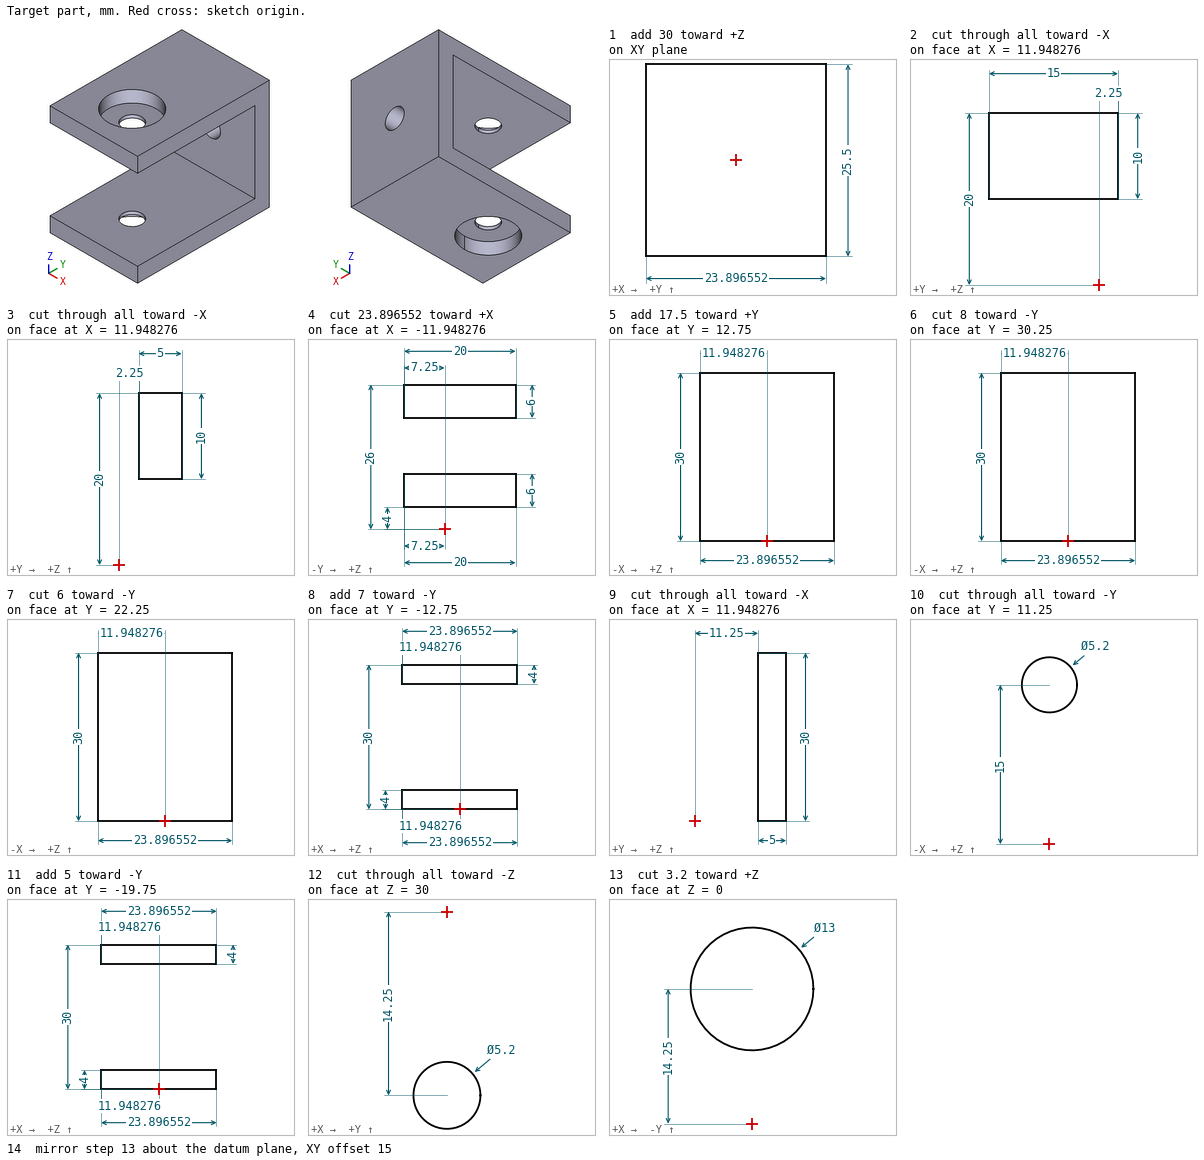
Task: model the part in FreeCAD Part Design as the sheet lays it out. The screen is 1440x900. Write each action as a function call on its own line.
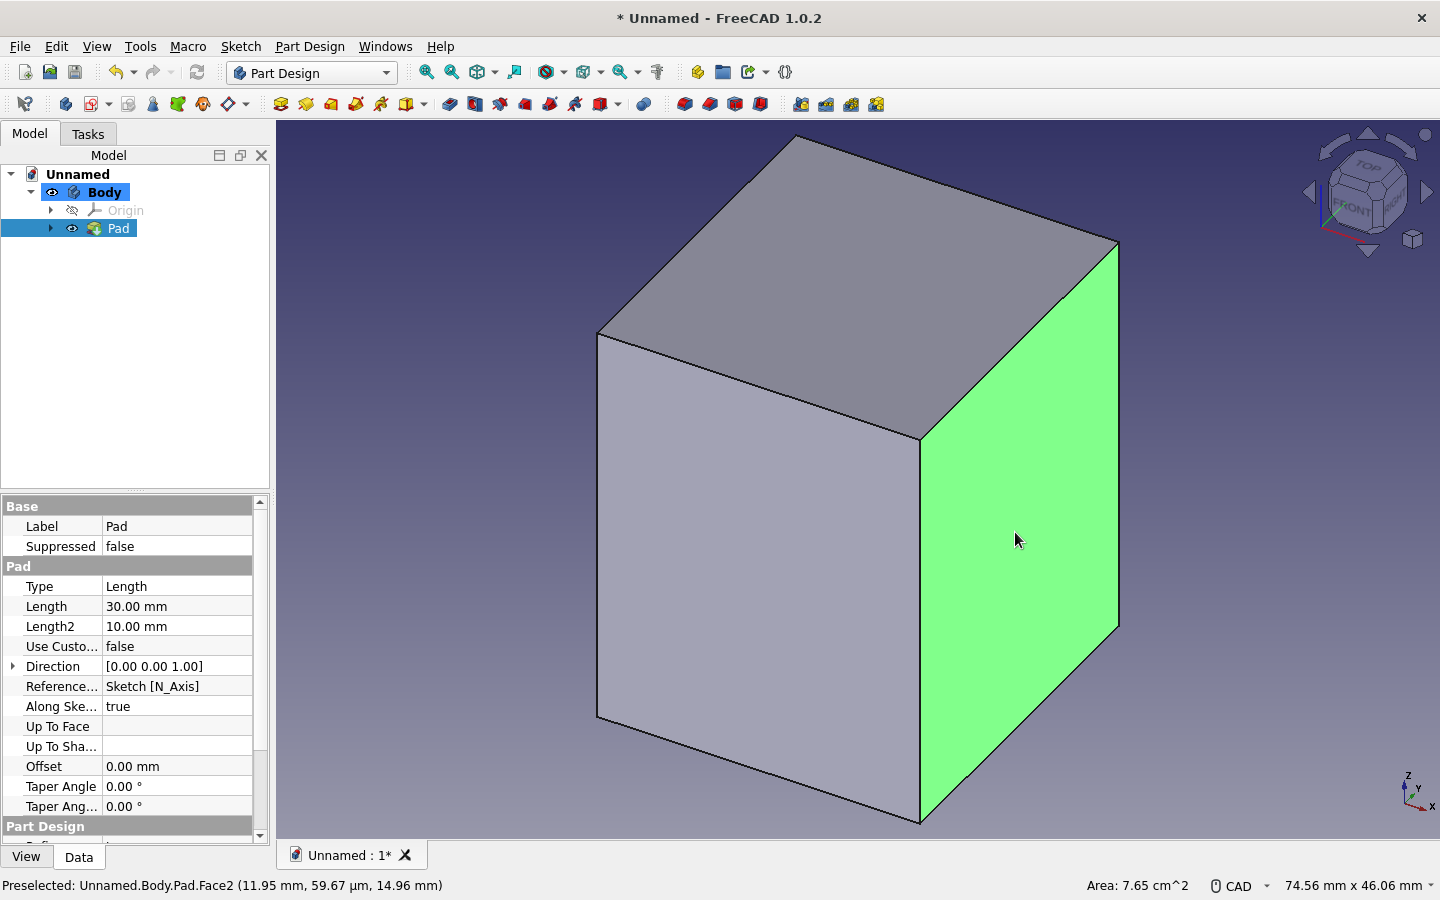
click(90, 104)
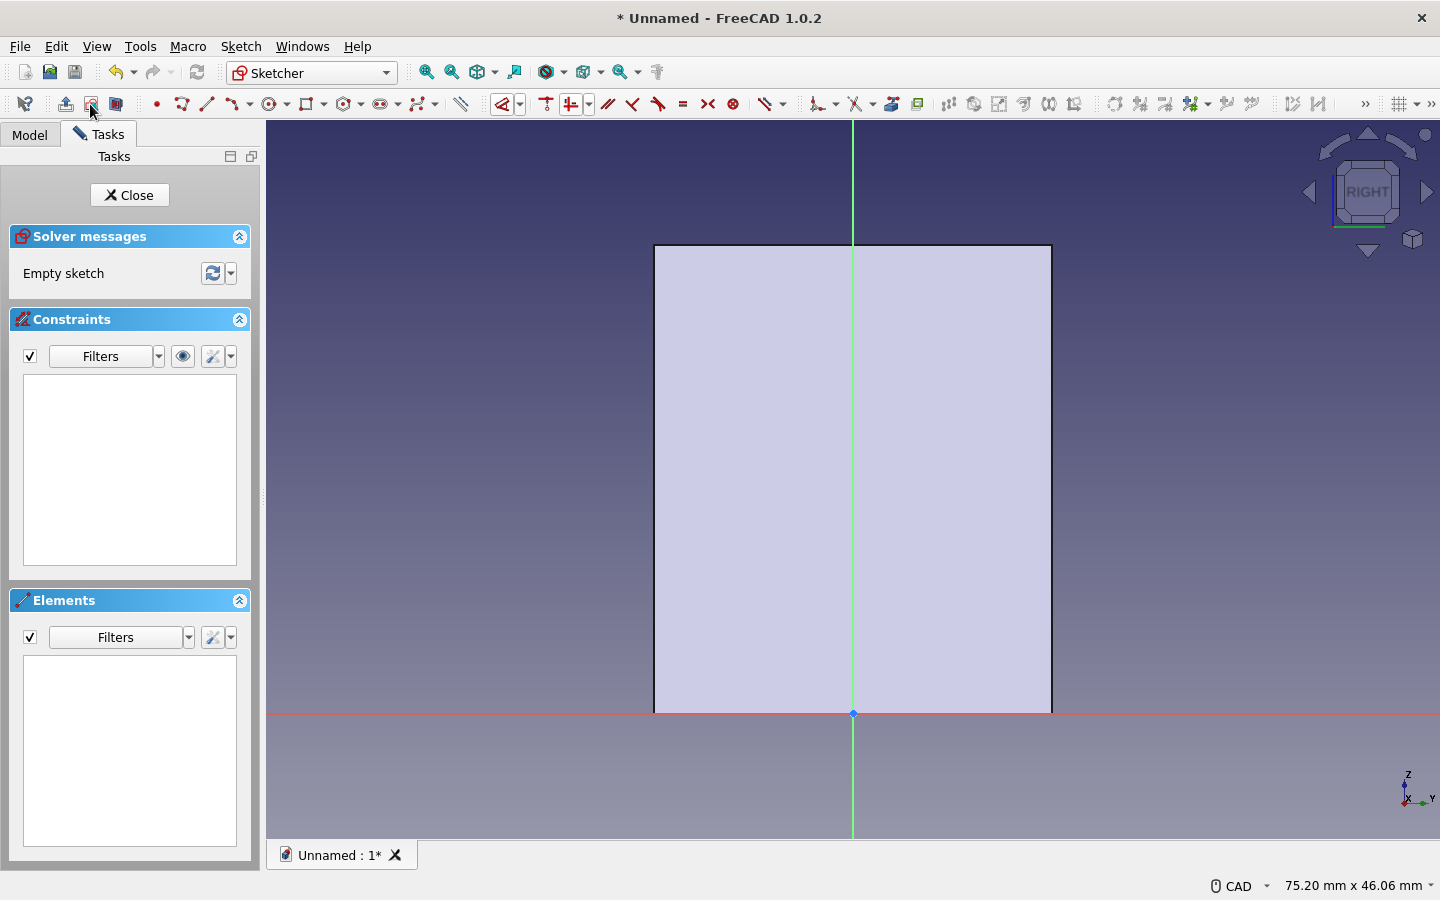
scroll(744, 716, up, 2)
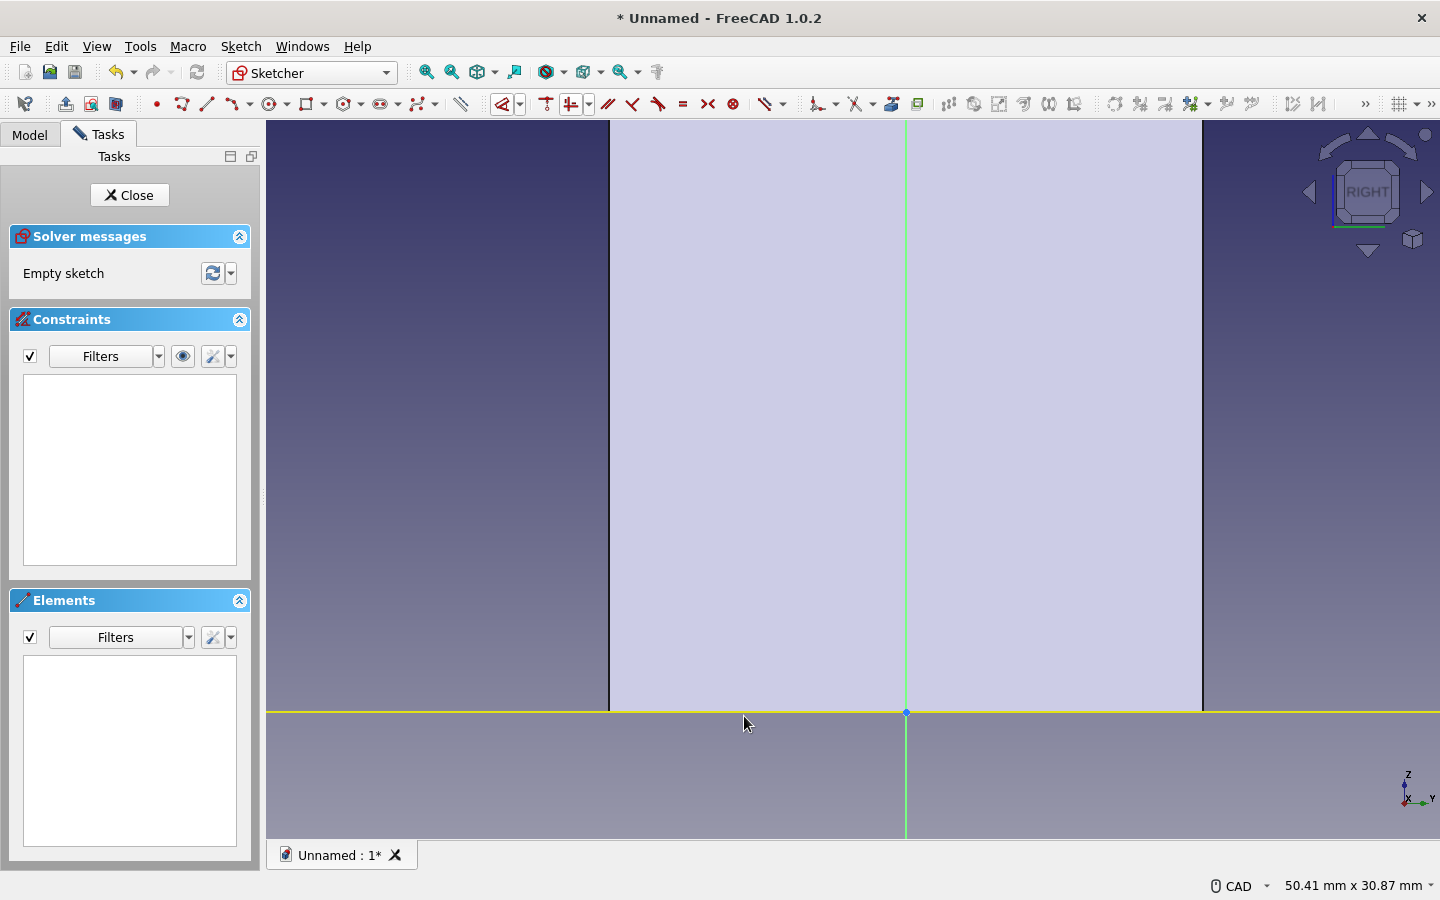
click(306, 104)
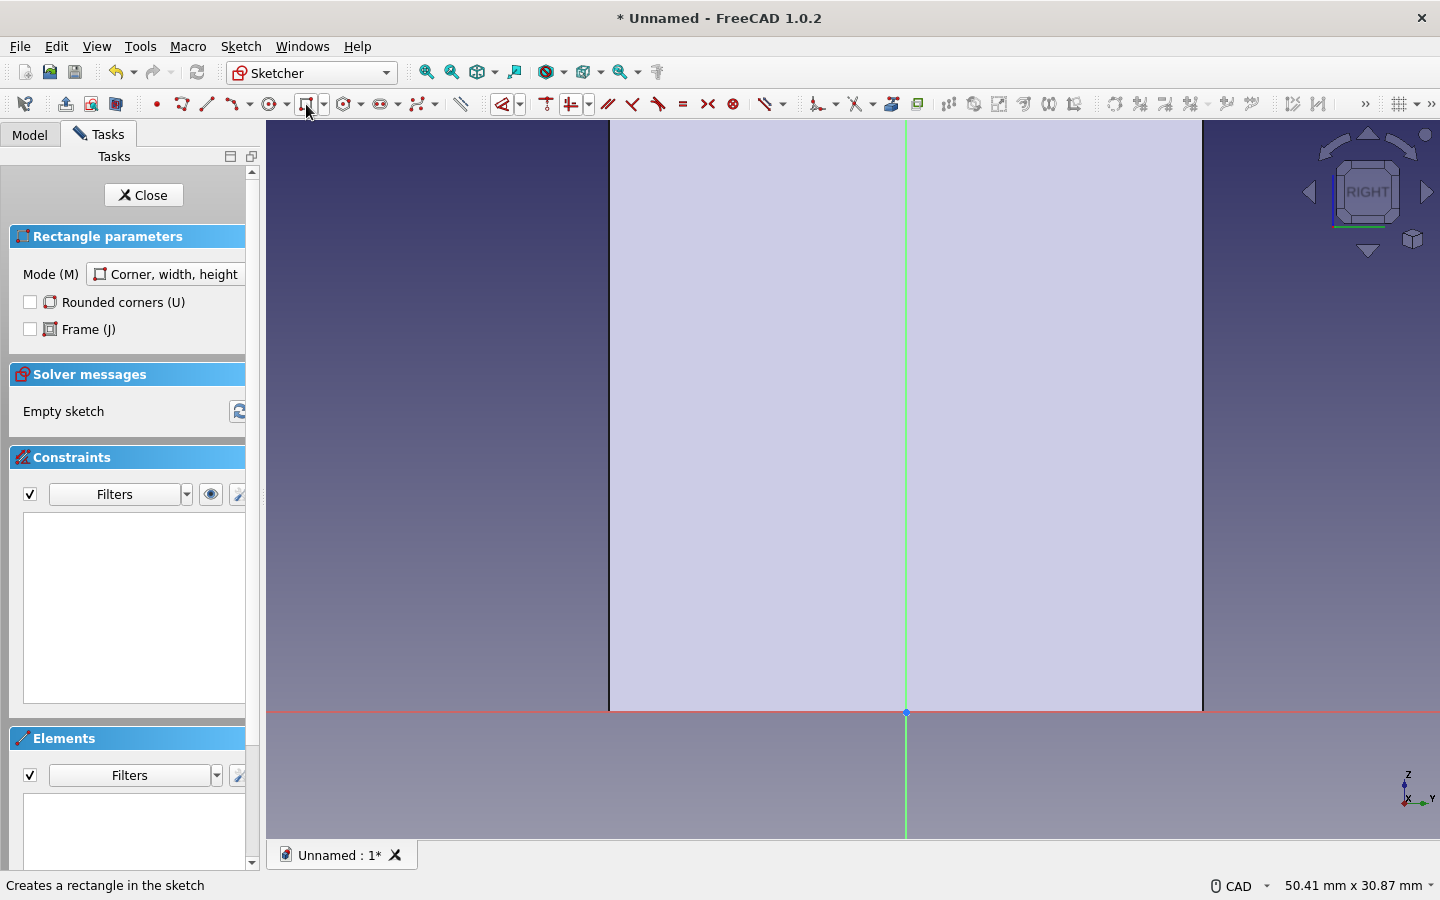
click(609, 246)
move(959, 479)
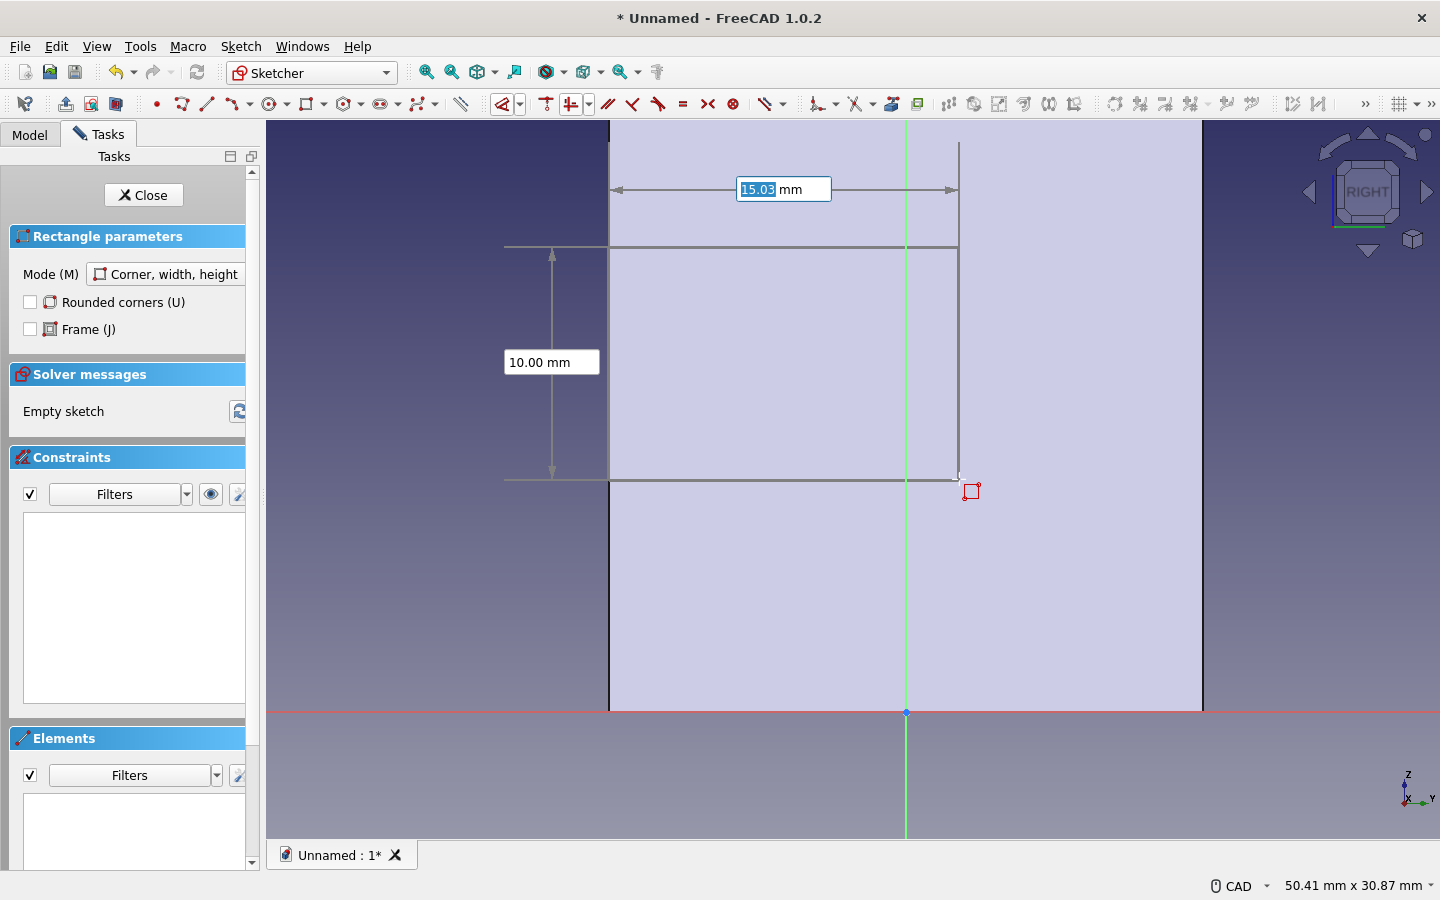
text(15)
key(Tab)
text(10)
key(Return)
key(Escape)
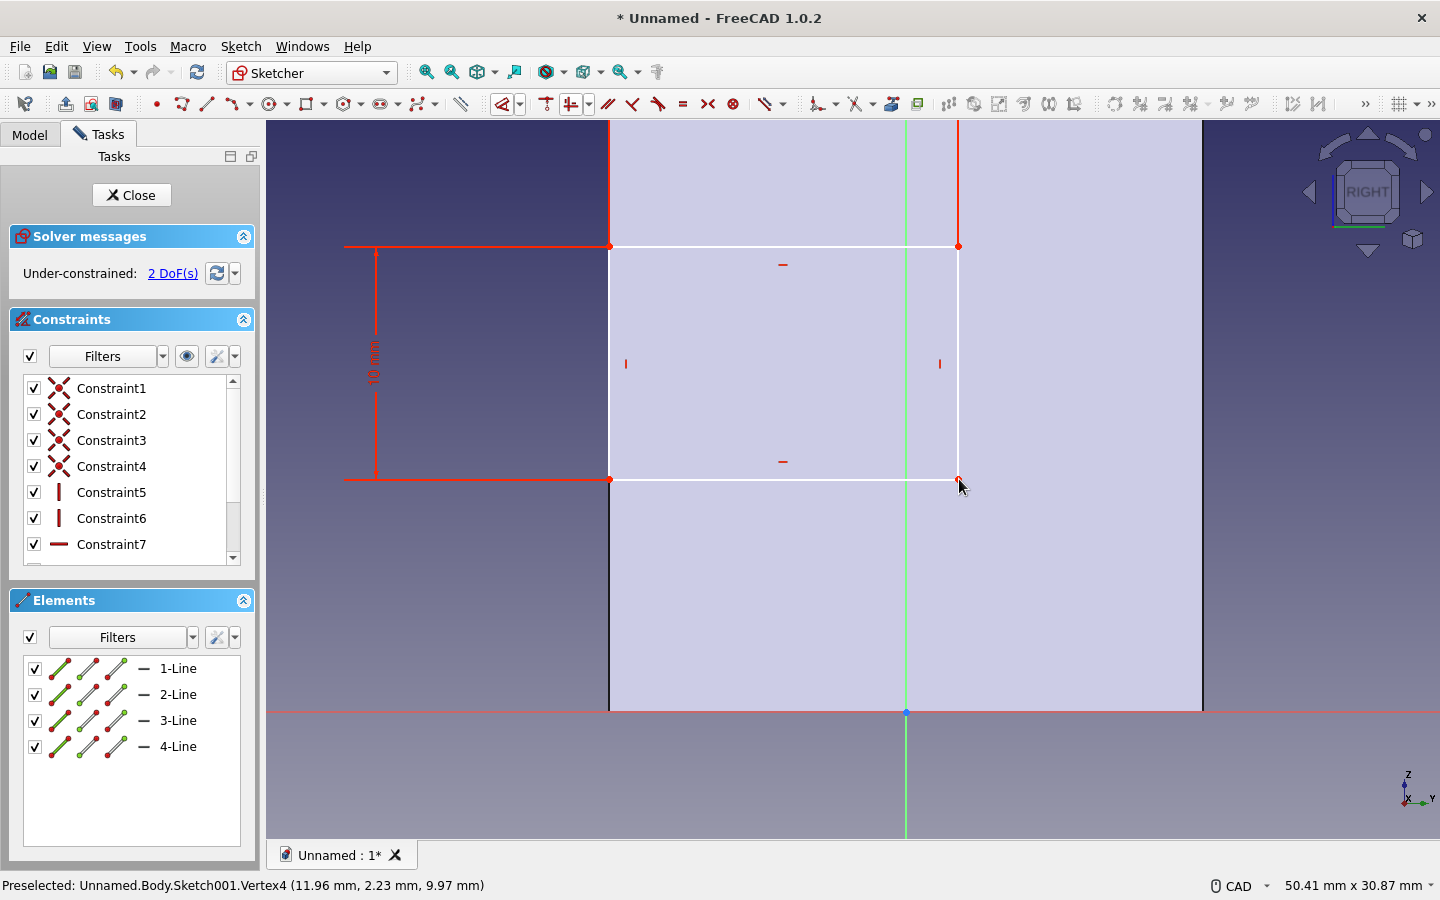
key(d)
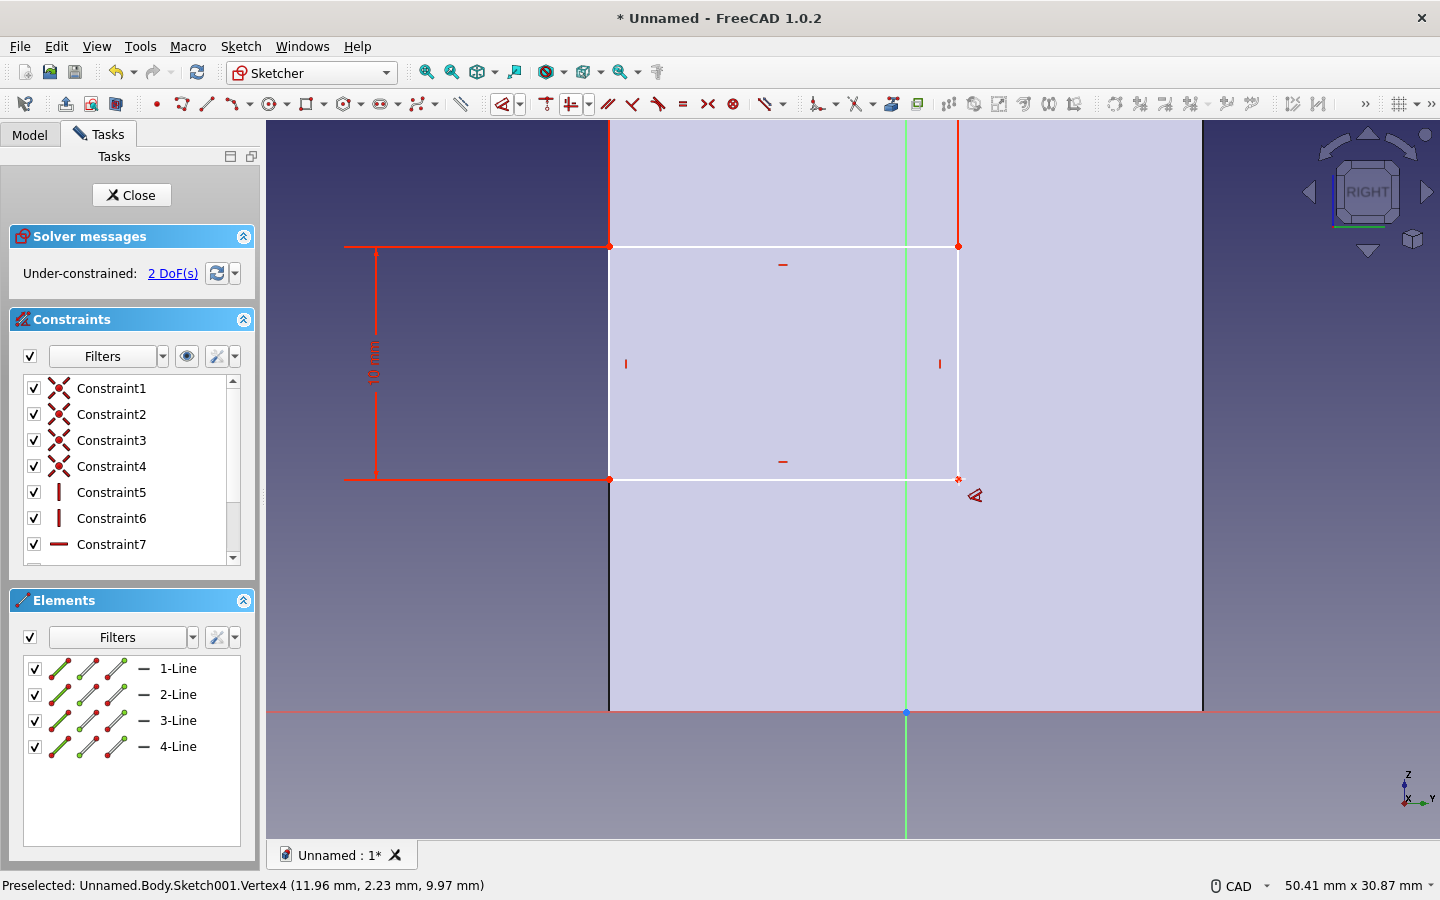
click(609, 247)
click(575, 480)